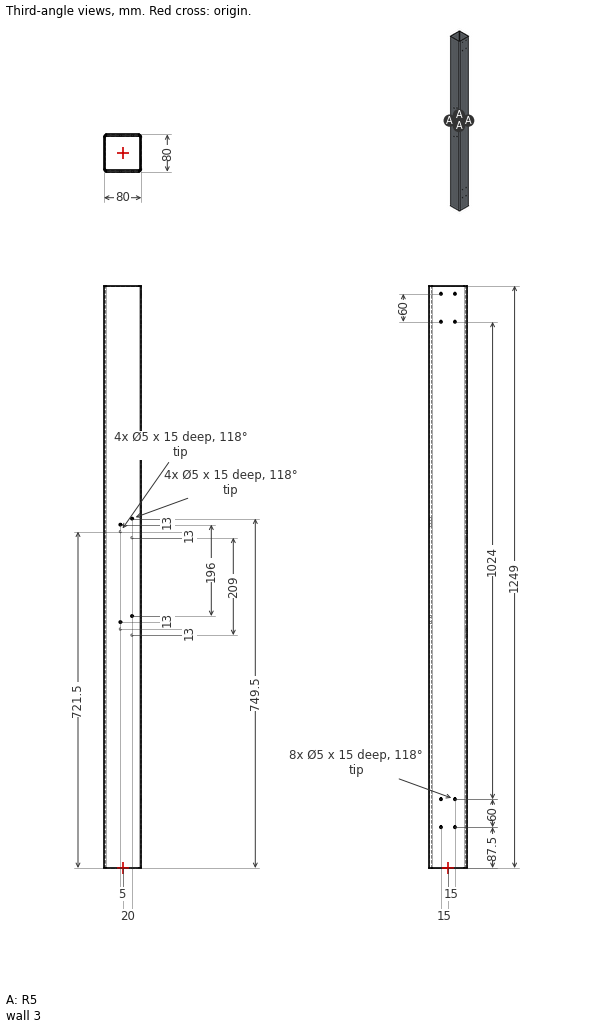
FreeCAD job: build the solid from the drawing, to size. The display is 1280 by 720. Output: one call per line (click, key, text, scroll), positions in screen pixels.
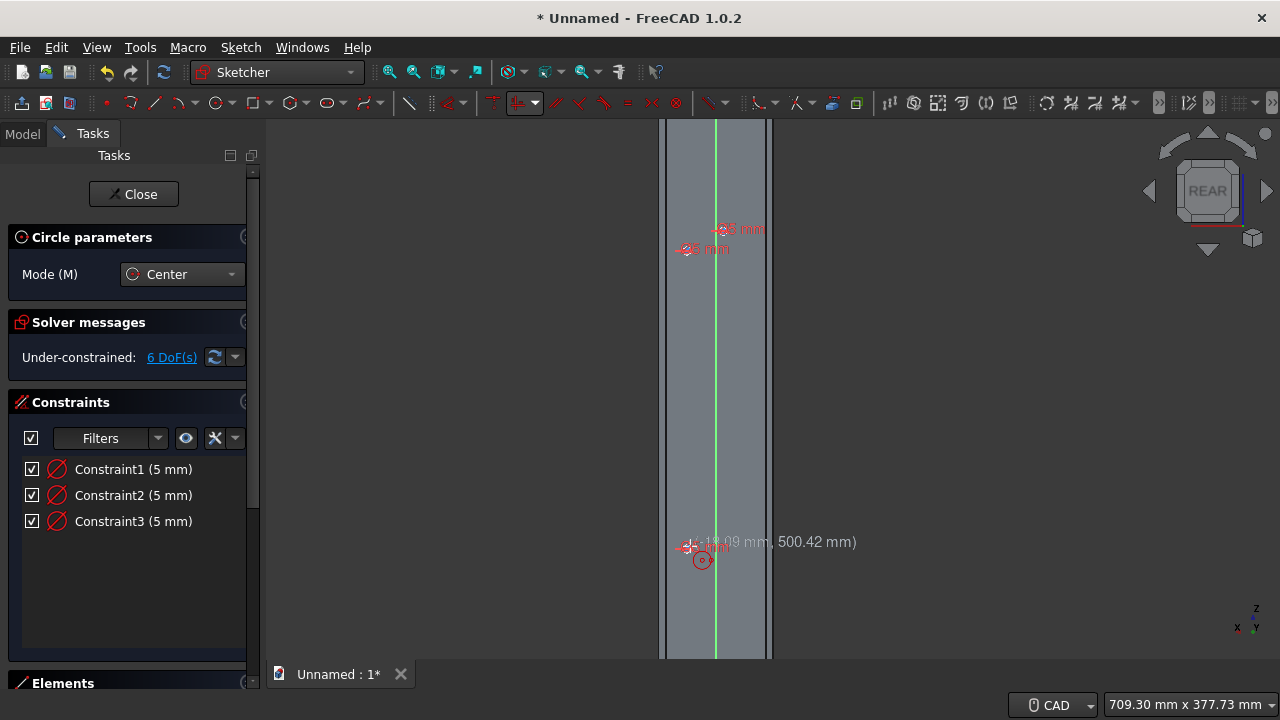
scroll(723, 530, up, 10)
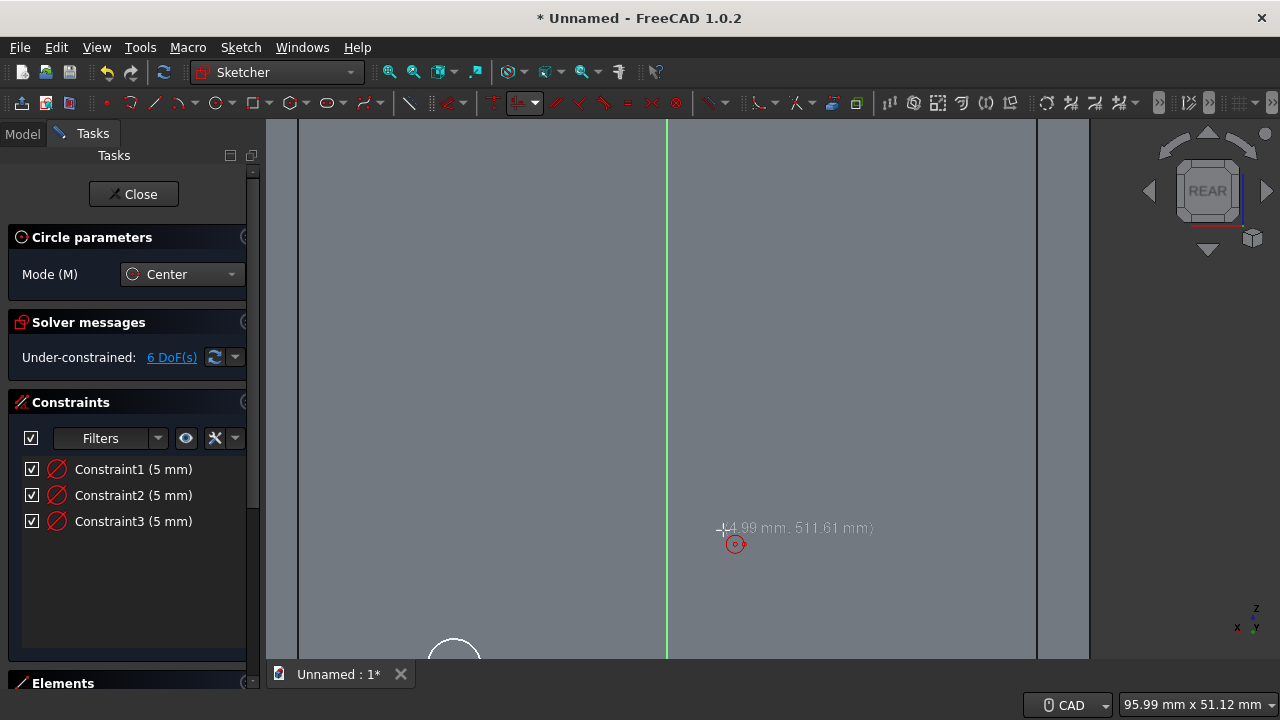
scroll(723, 530, down, 10)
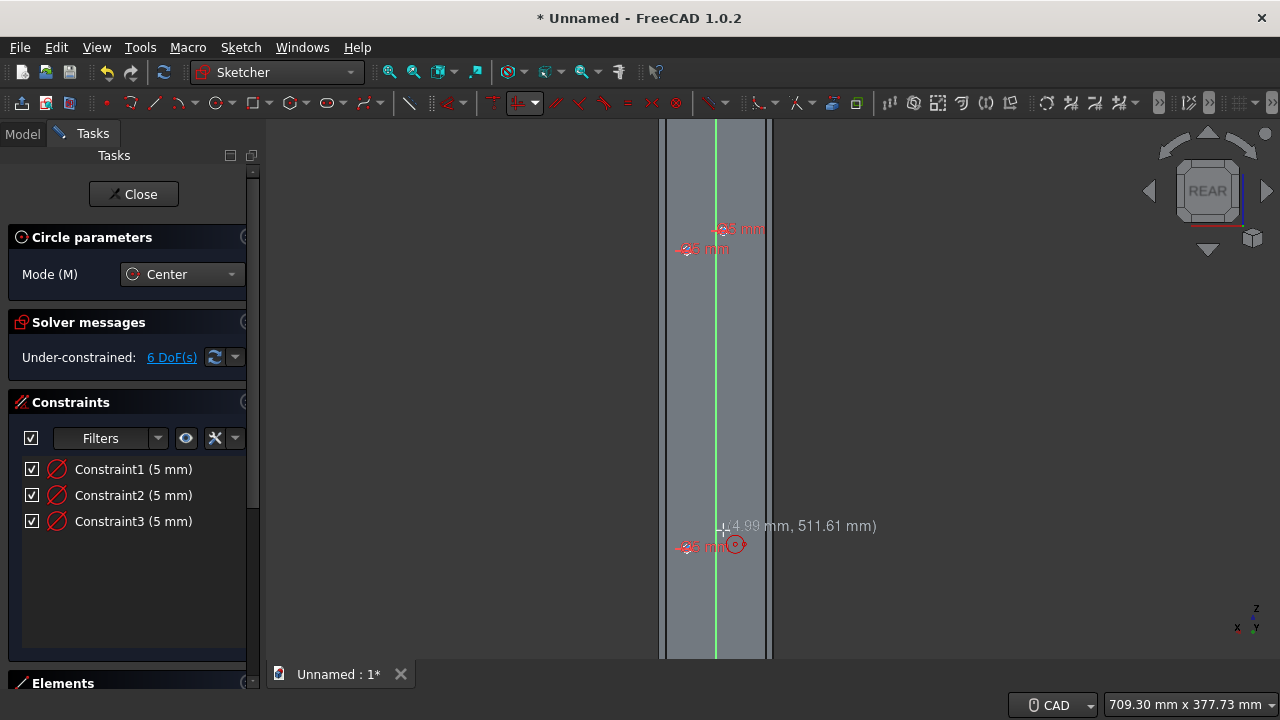
scroll(723, 530, up, 4)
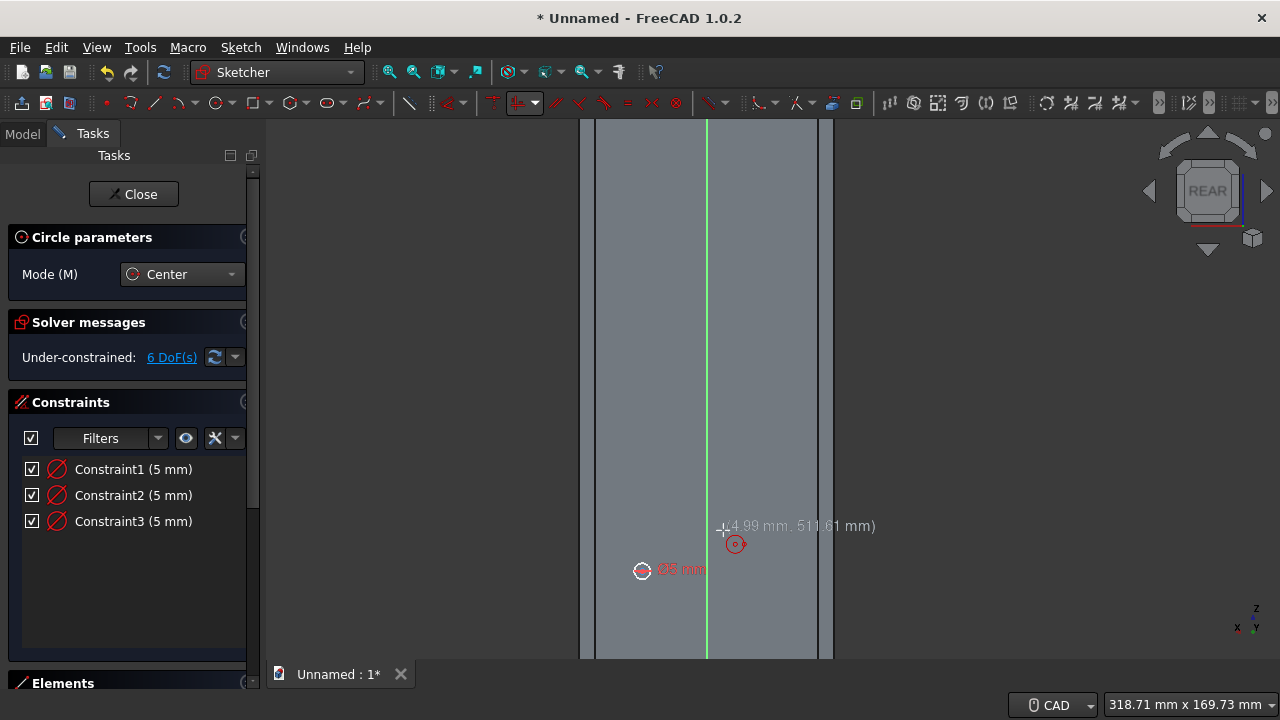
click(722, 528)
move(728, 523)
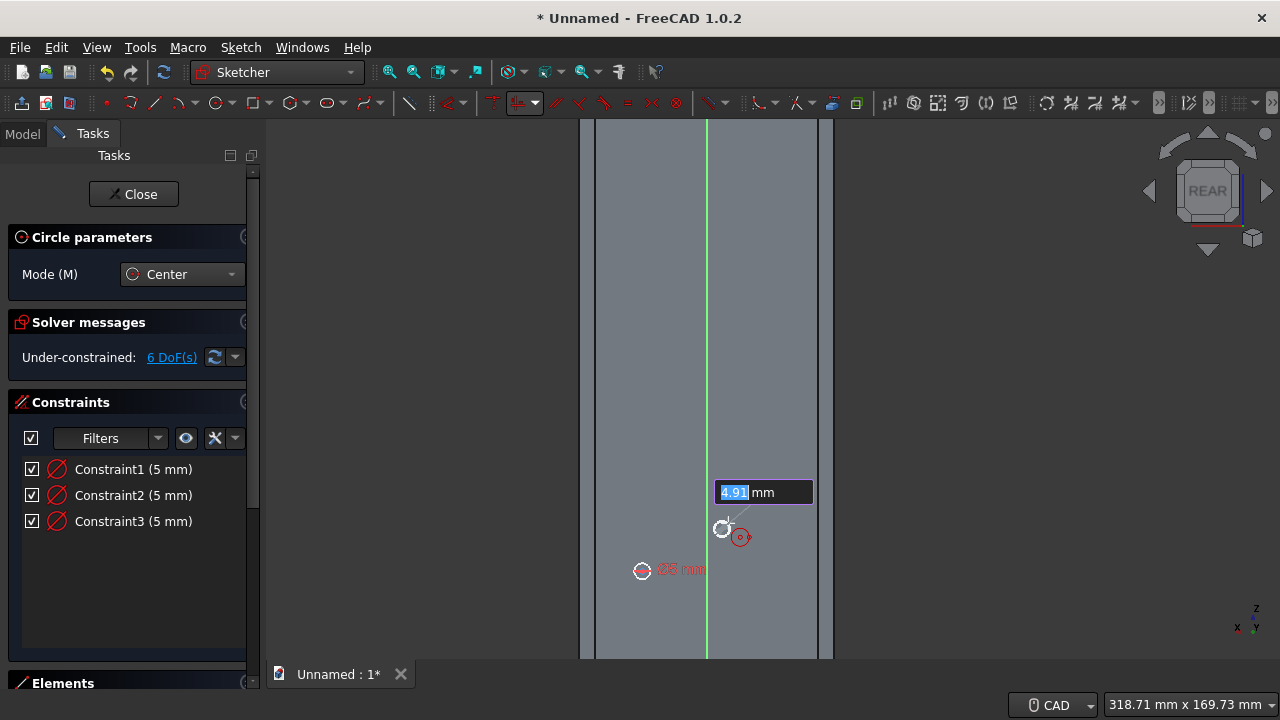
text(5)
key(Return)
key(Escape)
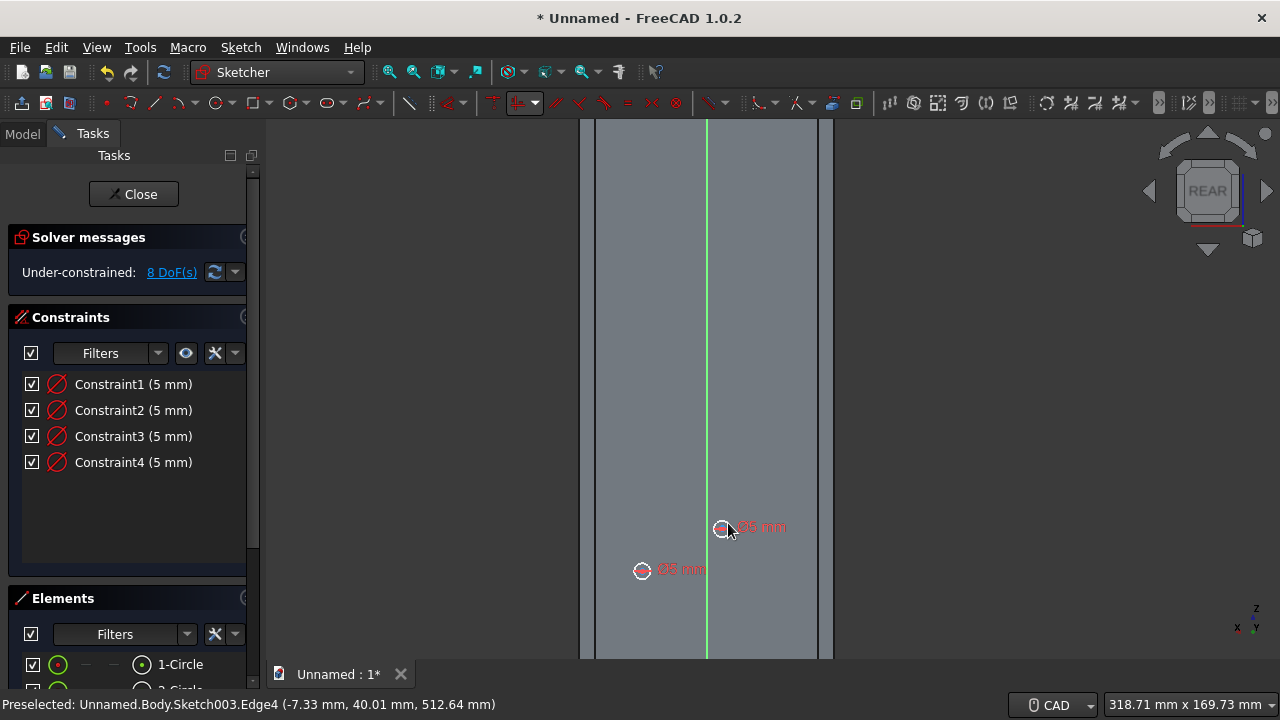
scroll(722, 530, down, 4)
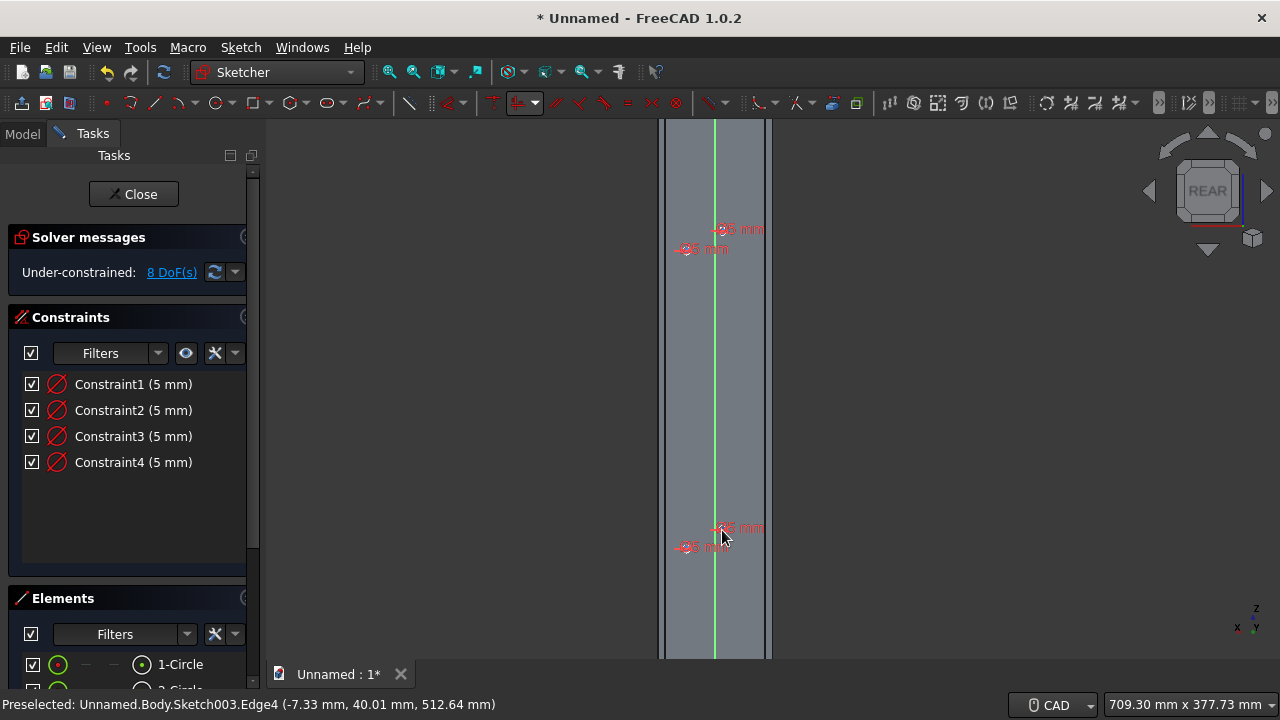
click(686, 251)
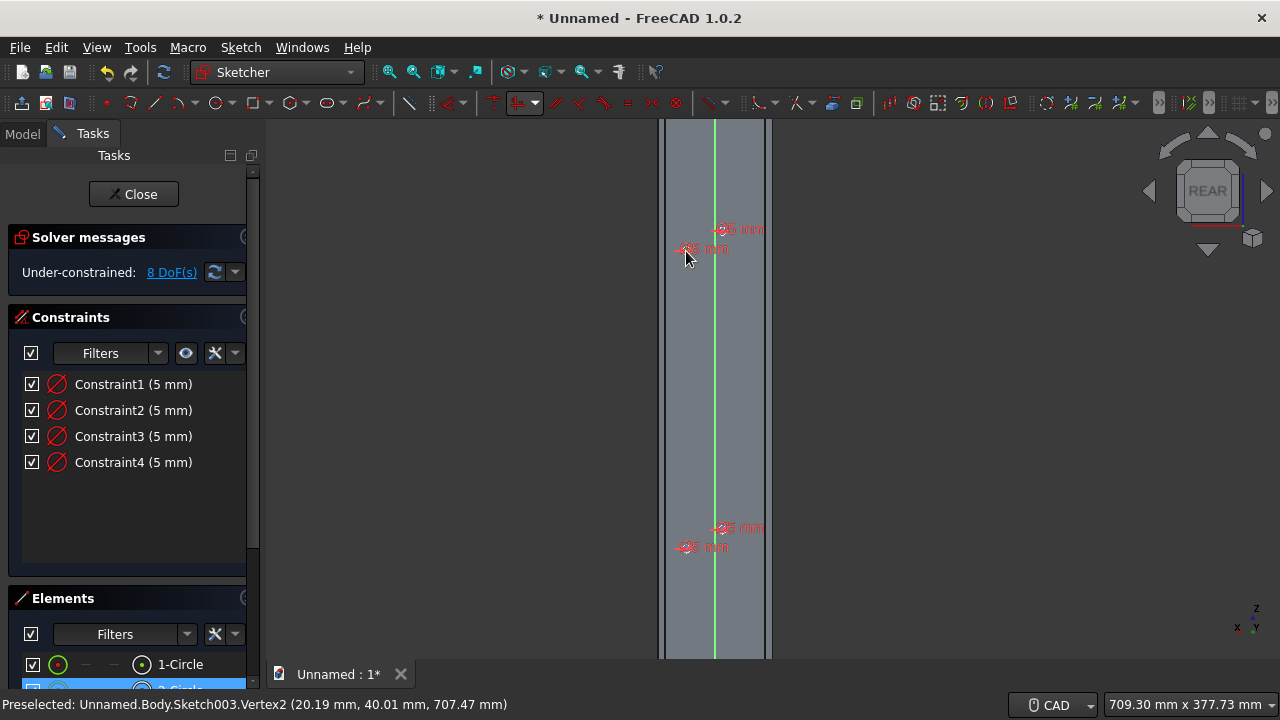
click(686, 549)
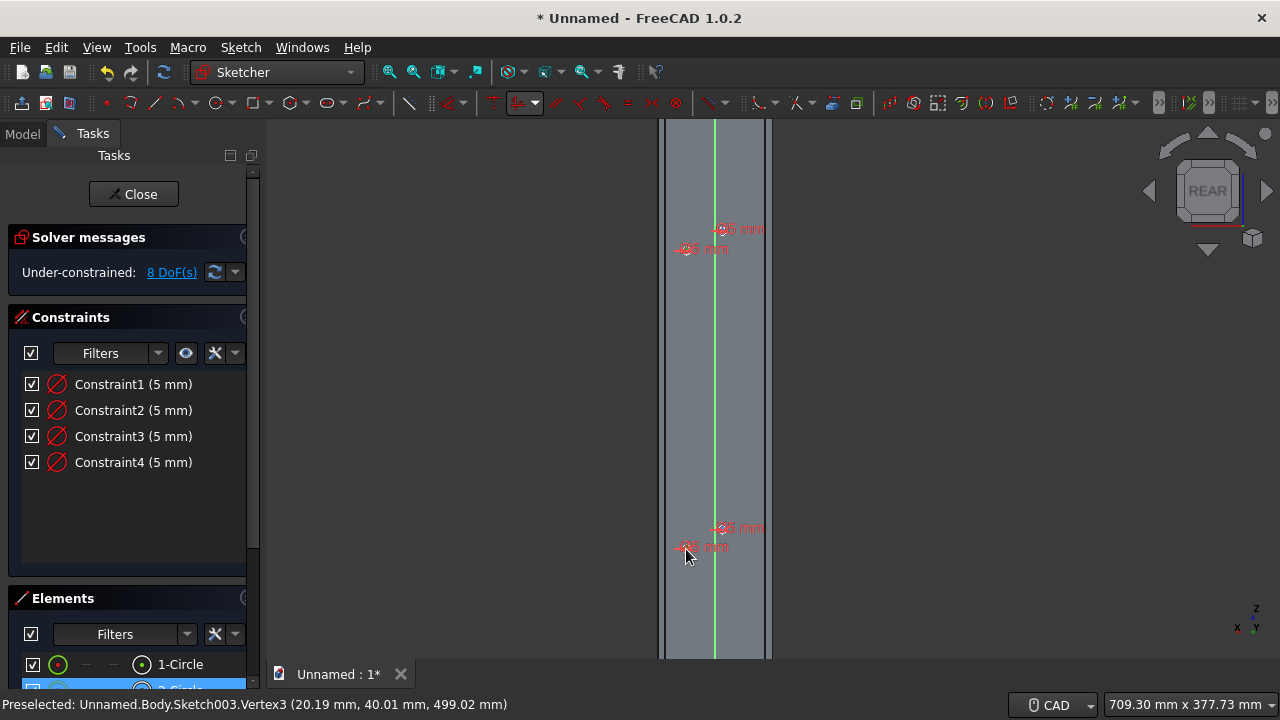
key(v)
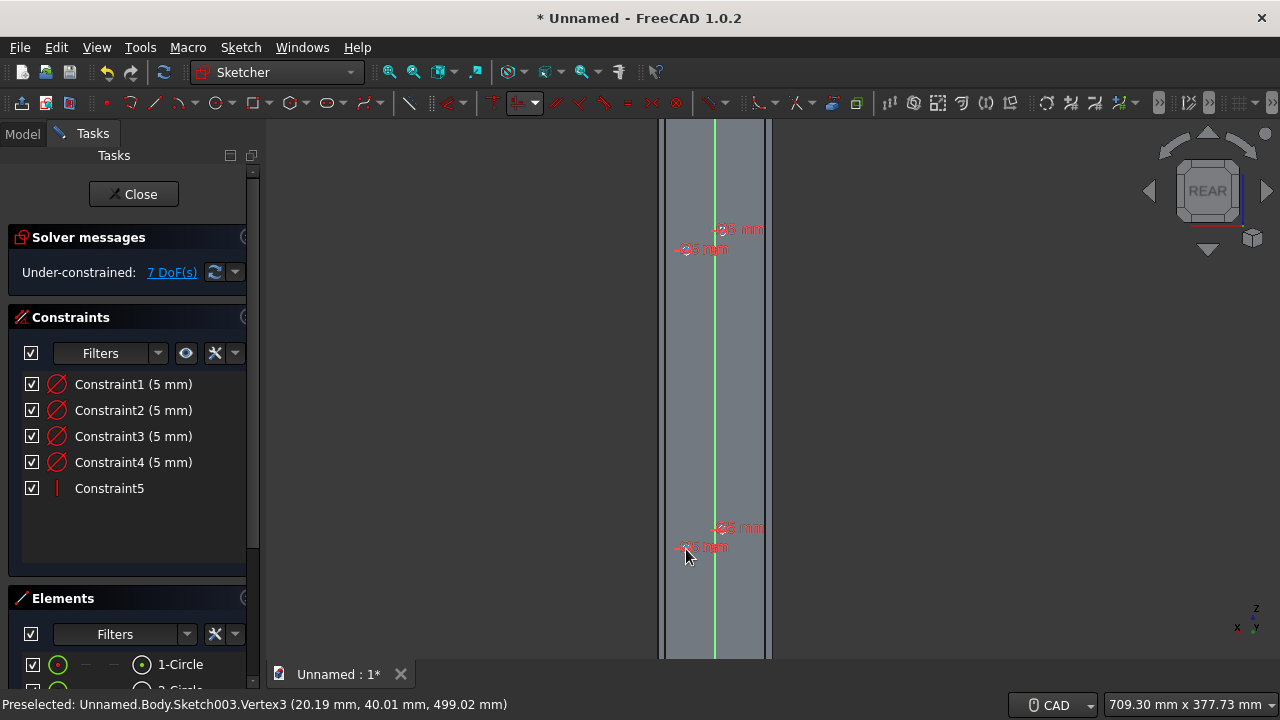
click(723, 231)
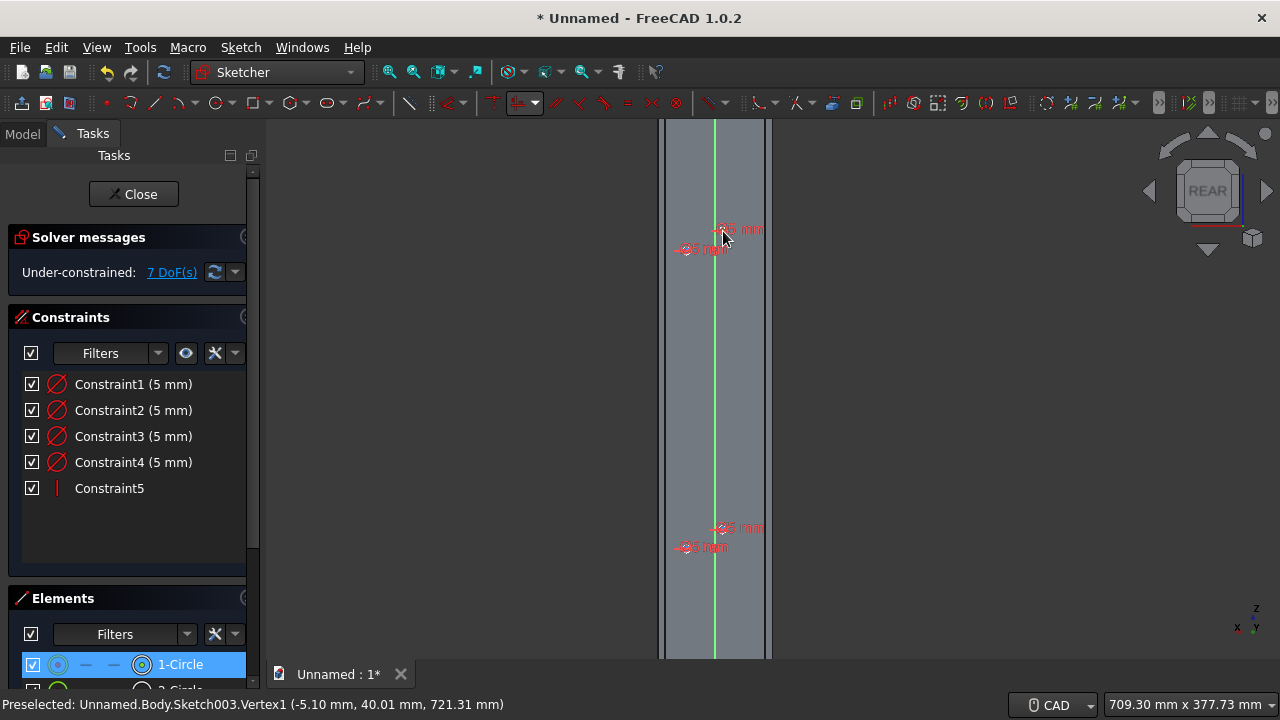
click(722, 530)